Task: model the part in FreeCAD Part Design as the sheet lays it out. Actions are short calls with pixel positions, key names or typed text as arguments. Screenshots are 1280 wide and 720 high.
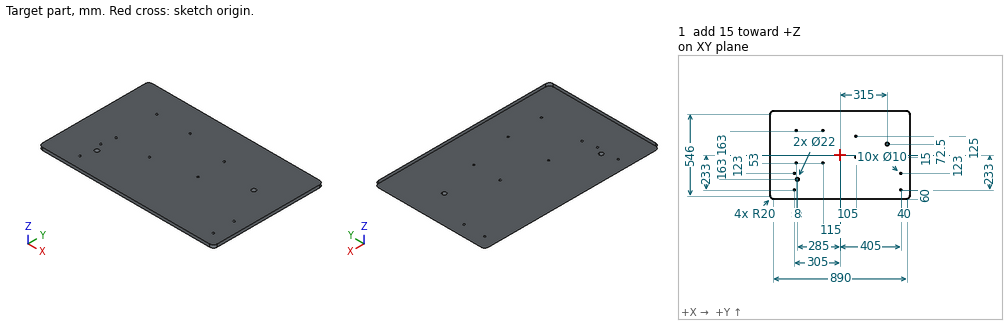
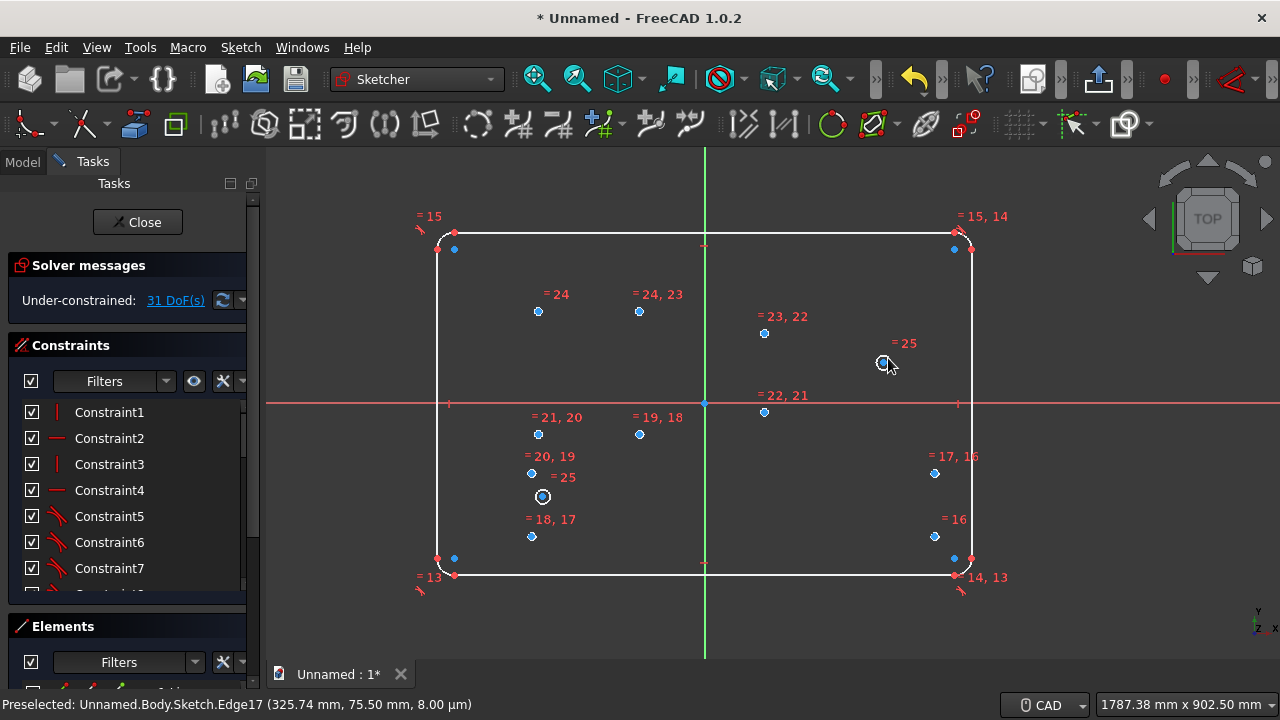
click(935, 537)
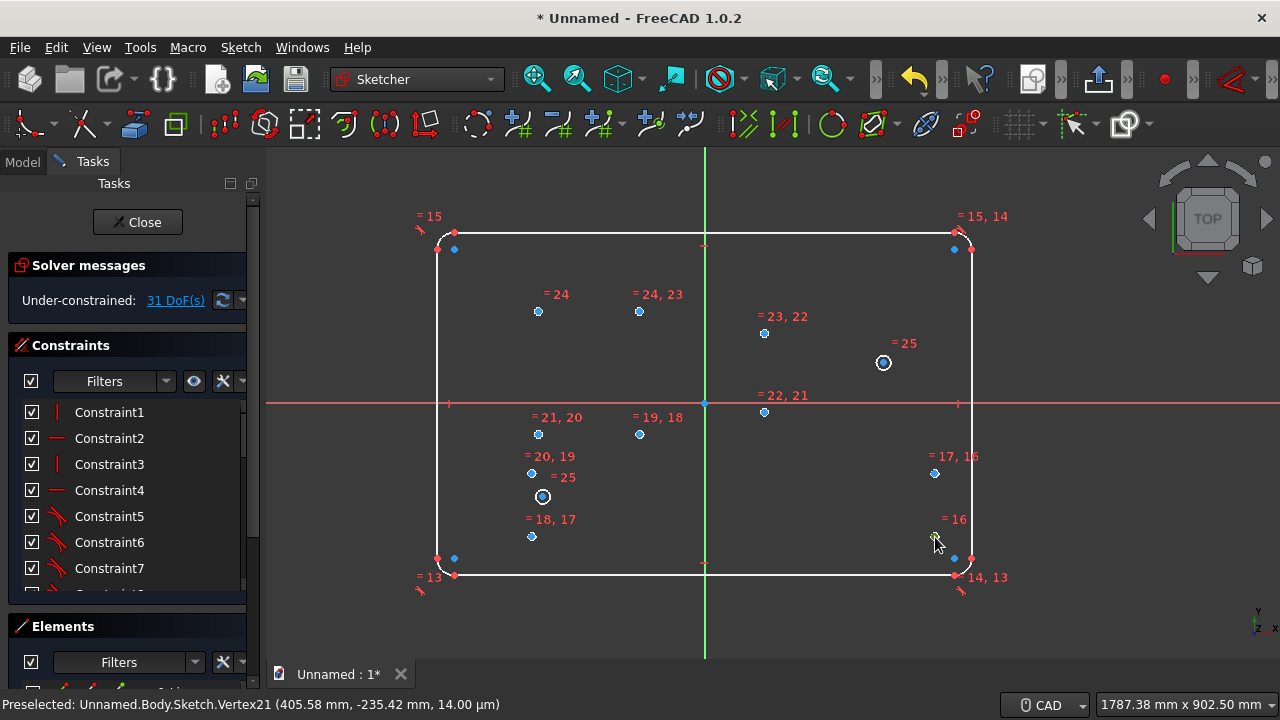
click(935, 474)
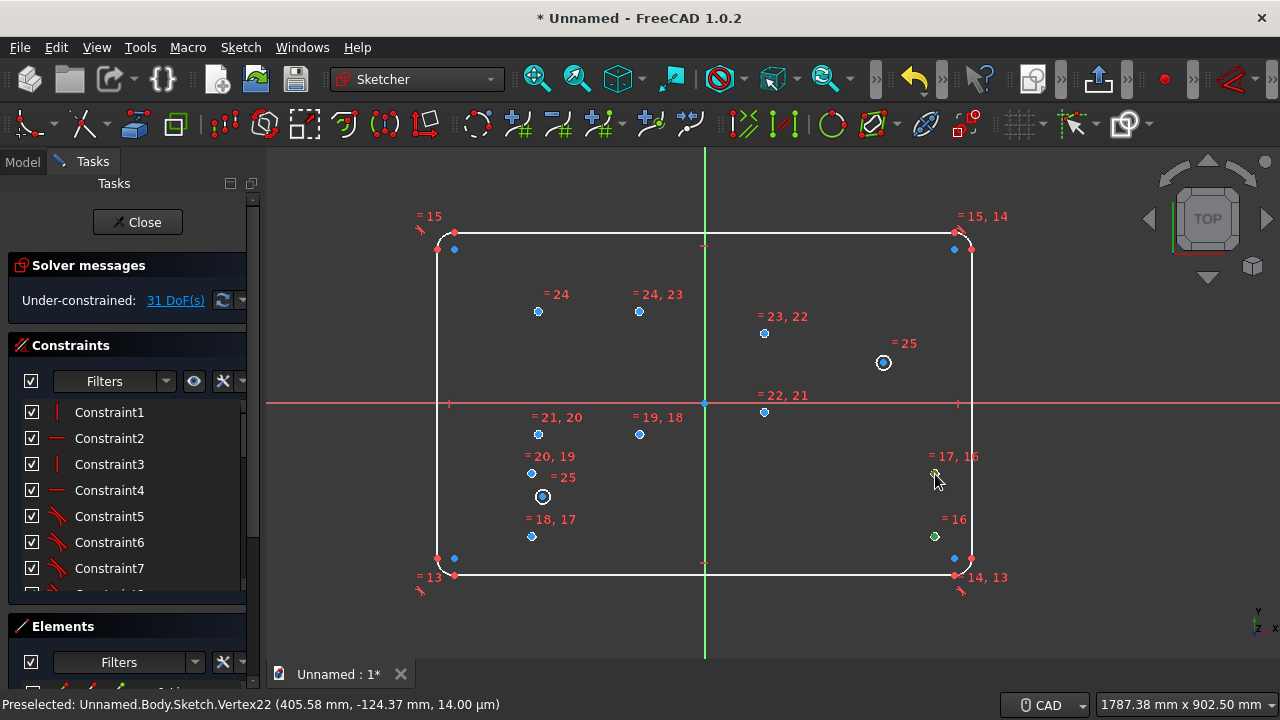
key(v)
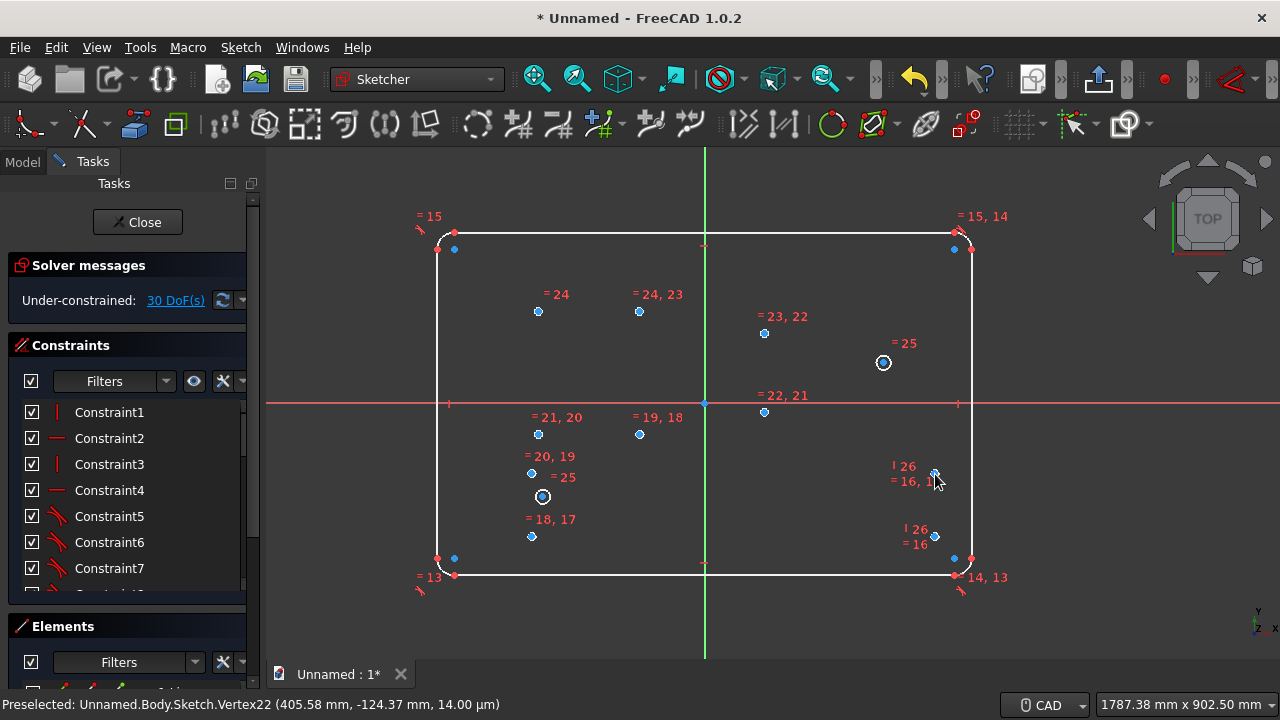
click(532, 537)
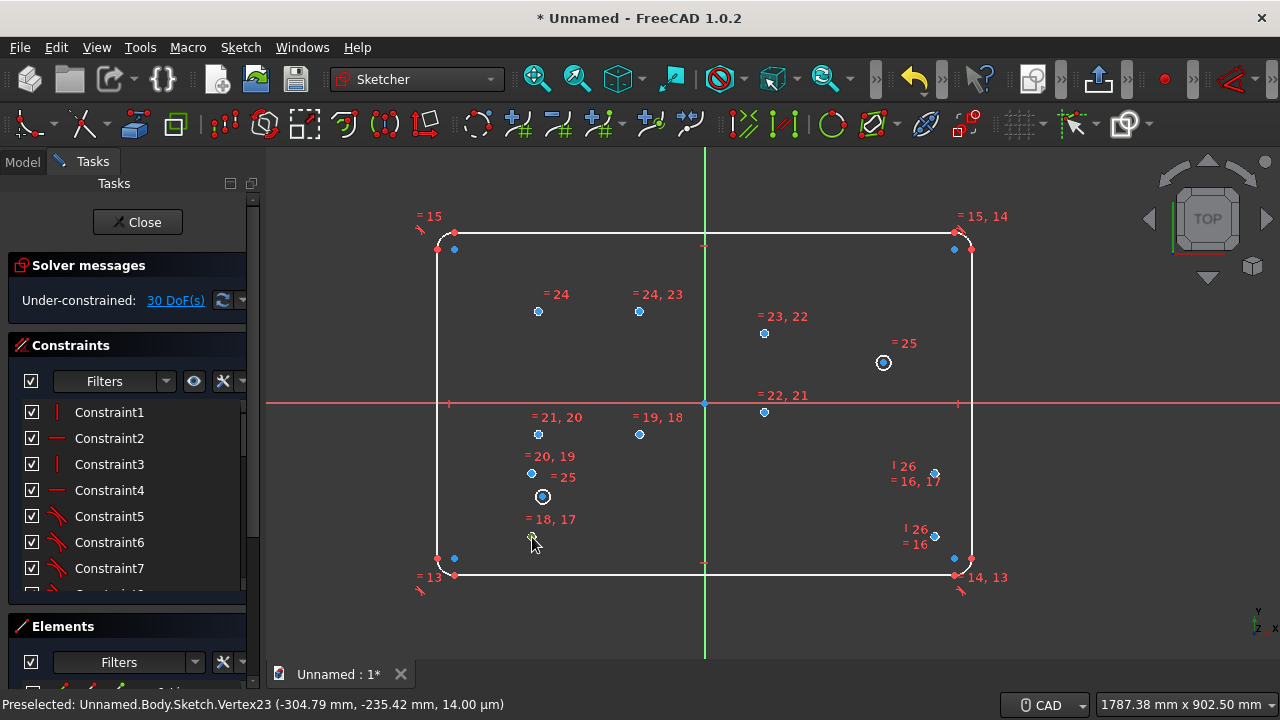
click(532, 474)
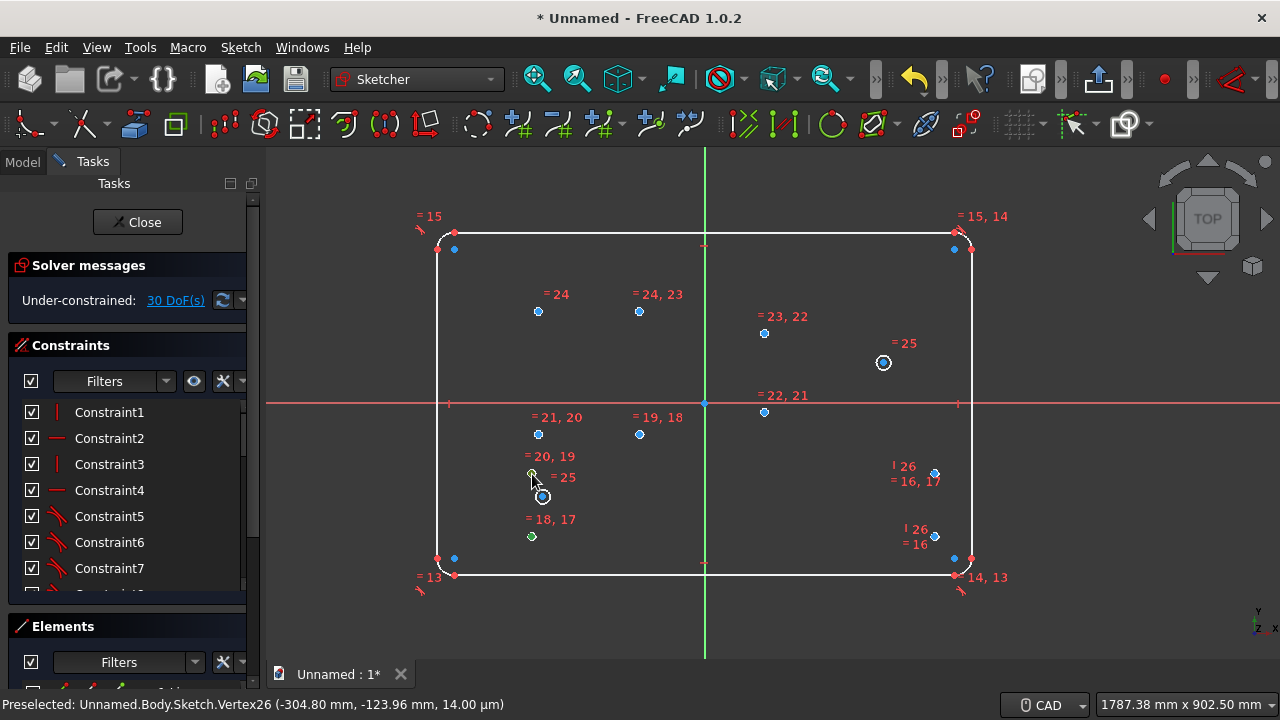
key(v)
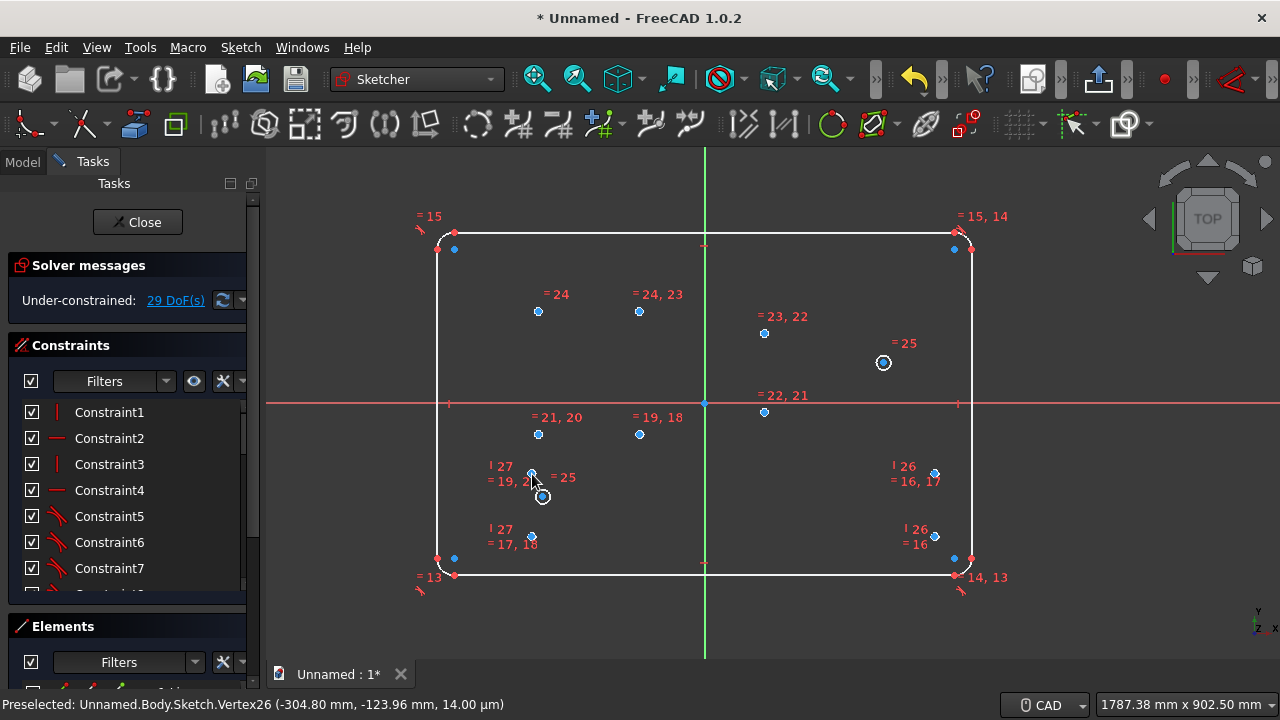
click(640, 435)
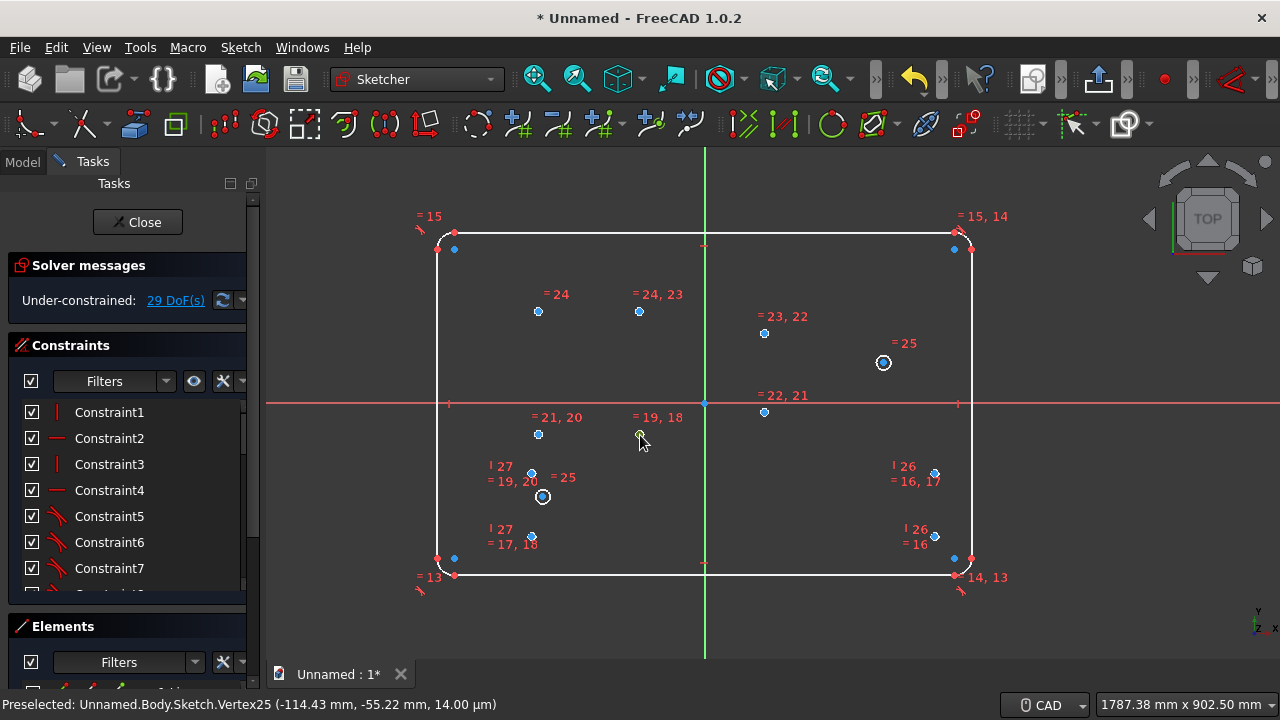
click(539, 434)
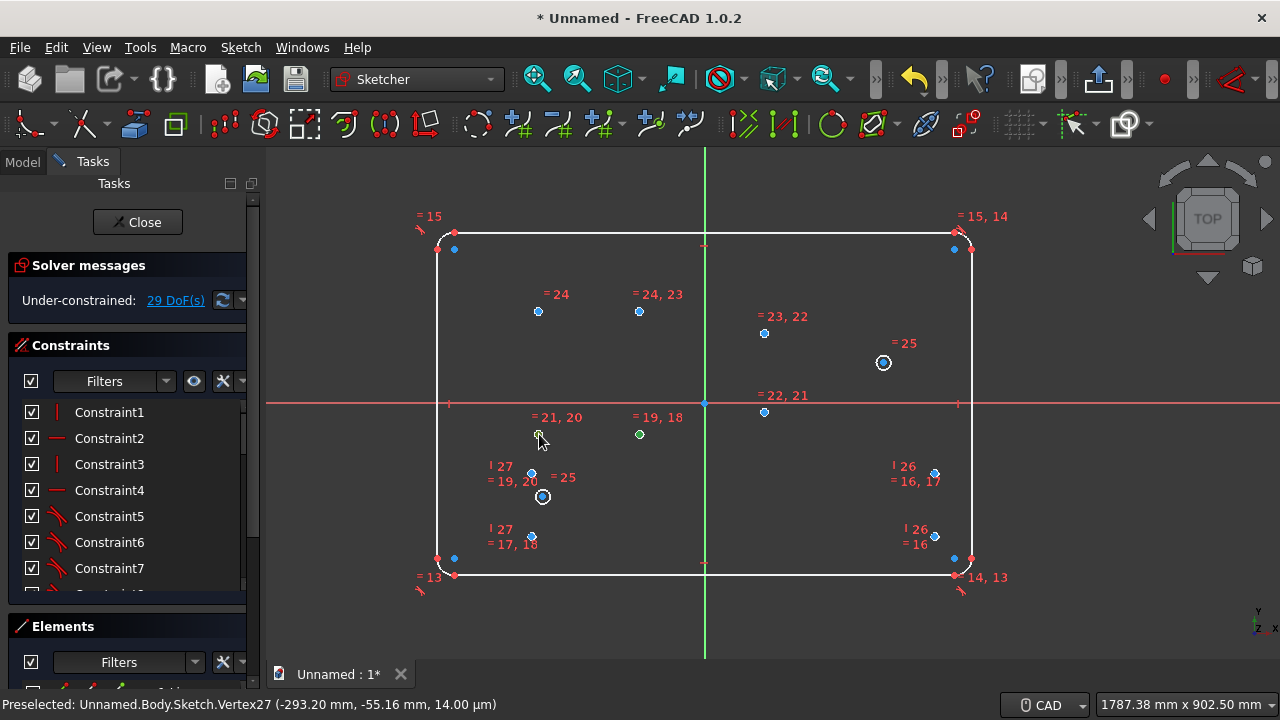
key(h)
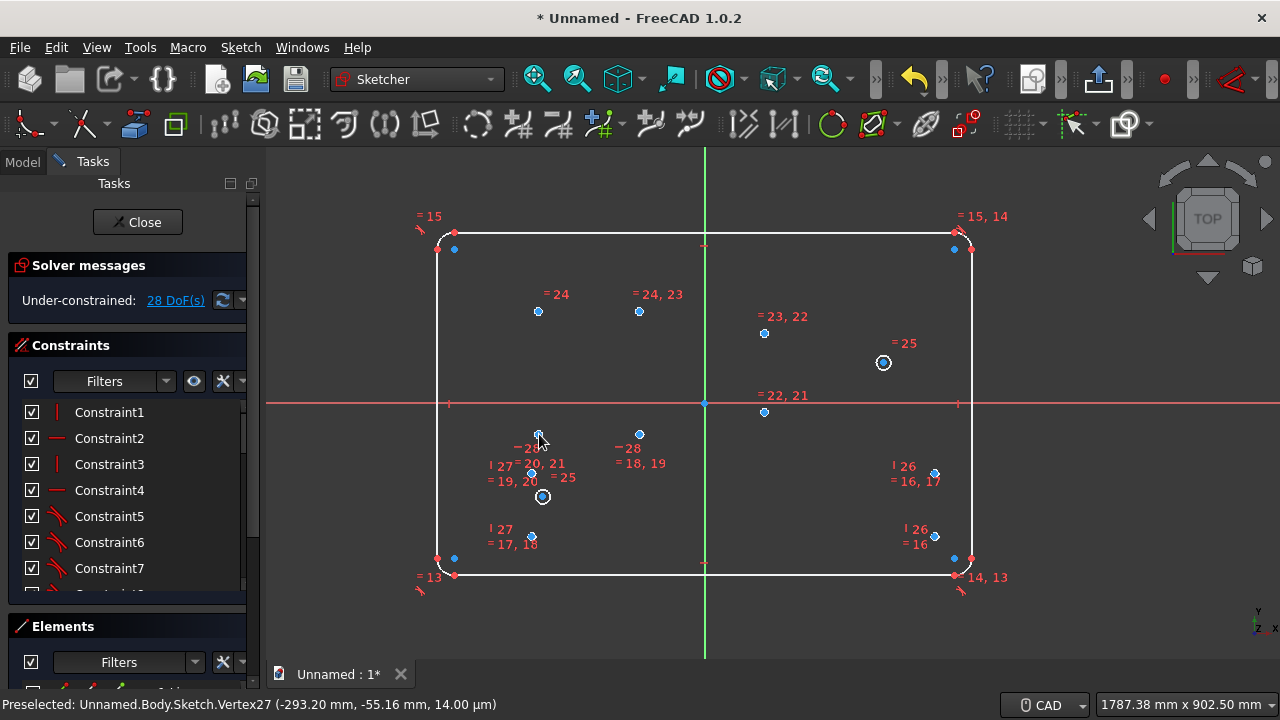
click(764, 412)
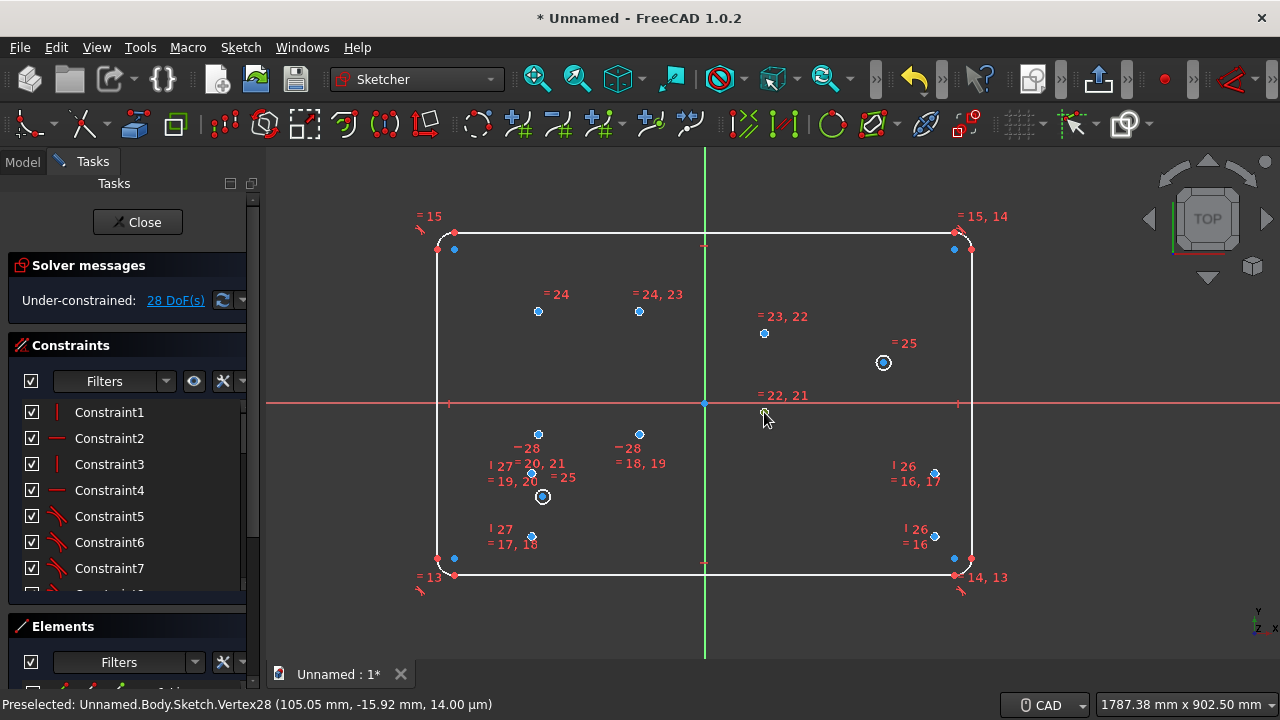
click(765, 334)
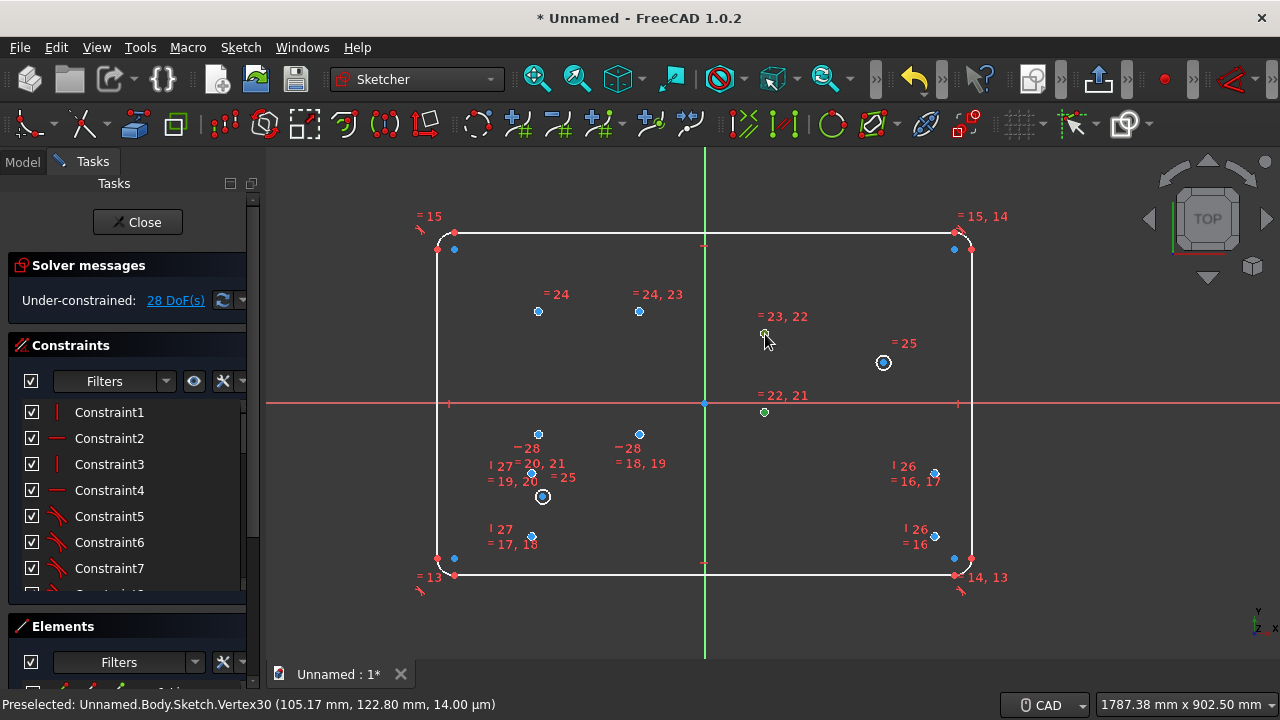
key(v)